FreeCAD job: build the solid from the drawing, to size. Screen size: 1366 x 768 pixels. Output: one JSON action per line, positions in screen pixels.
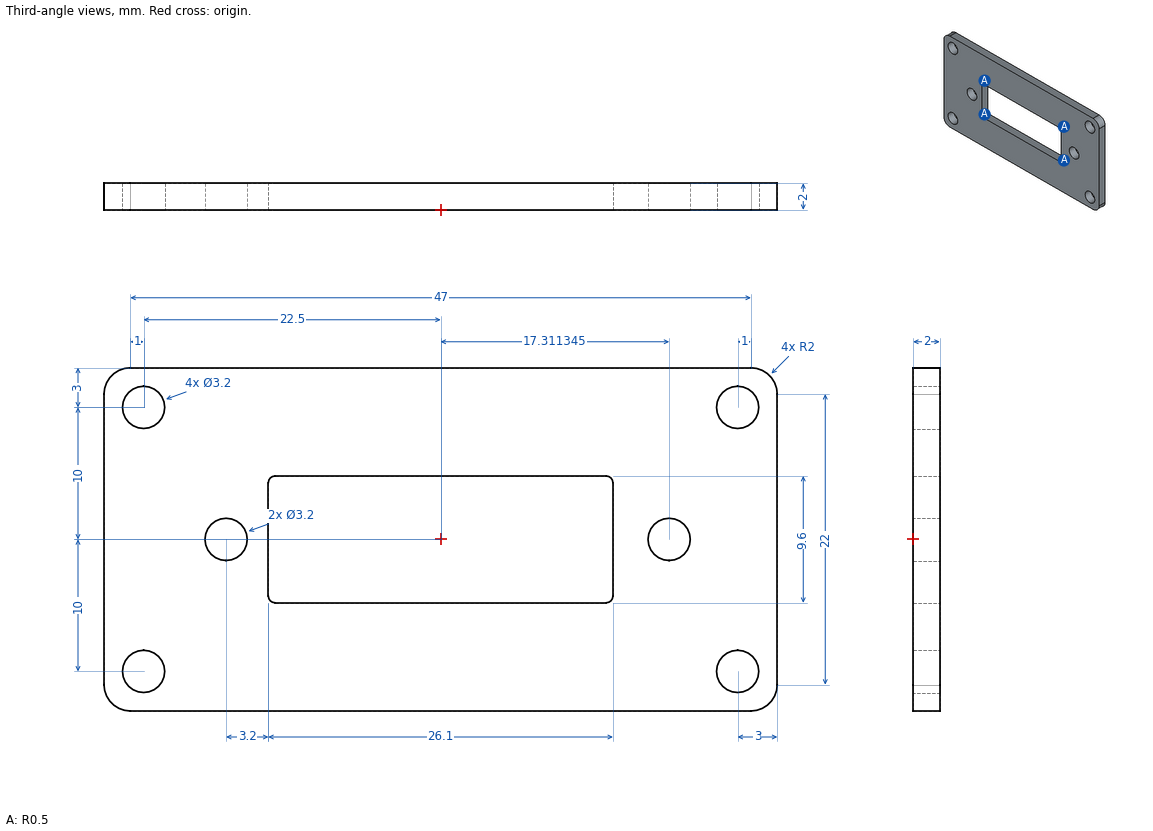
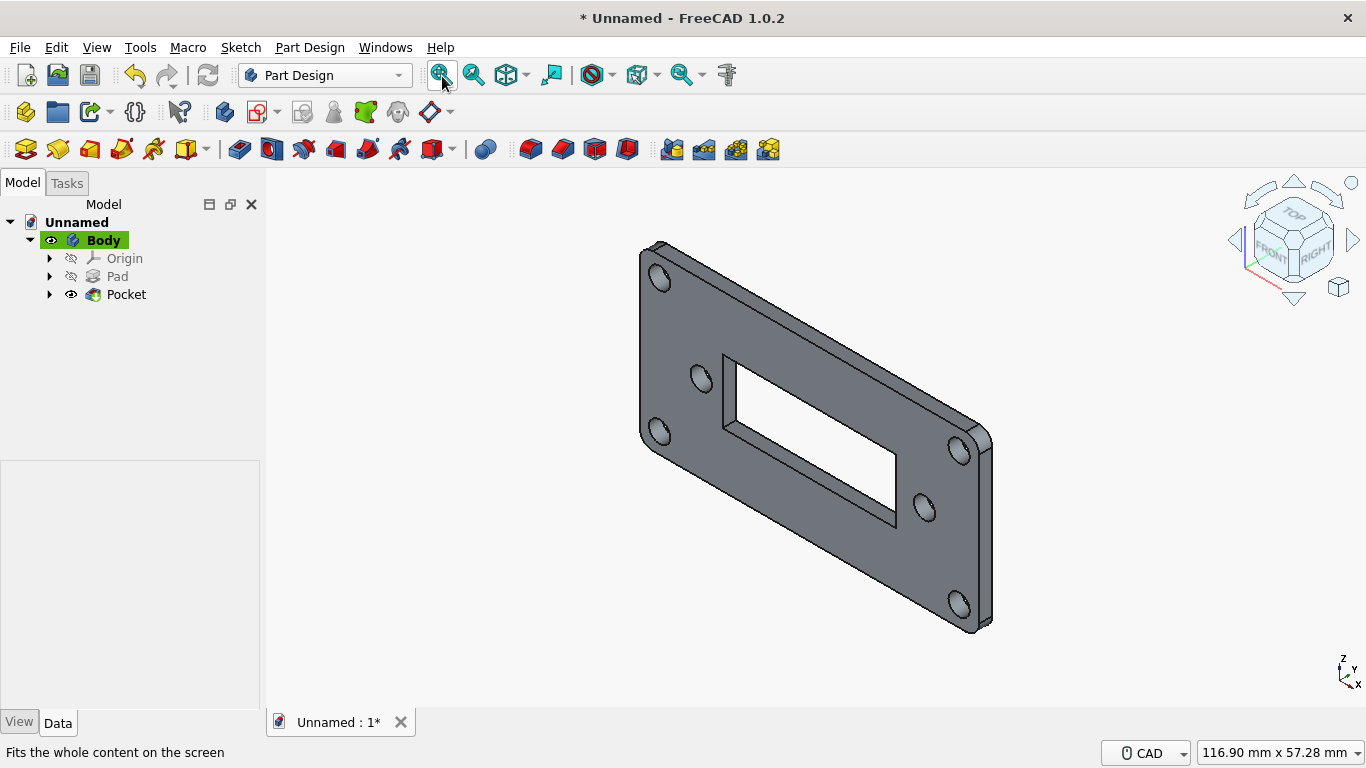
{"action": "scroll", "coordinate": [903, 450], "scroll_direction": "up", "scroll_amount": 4}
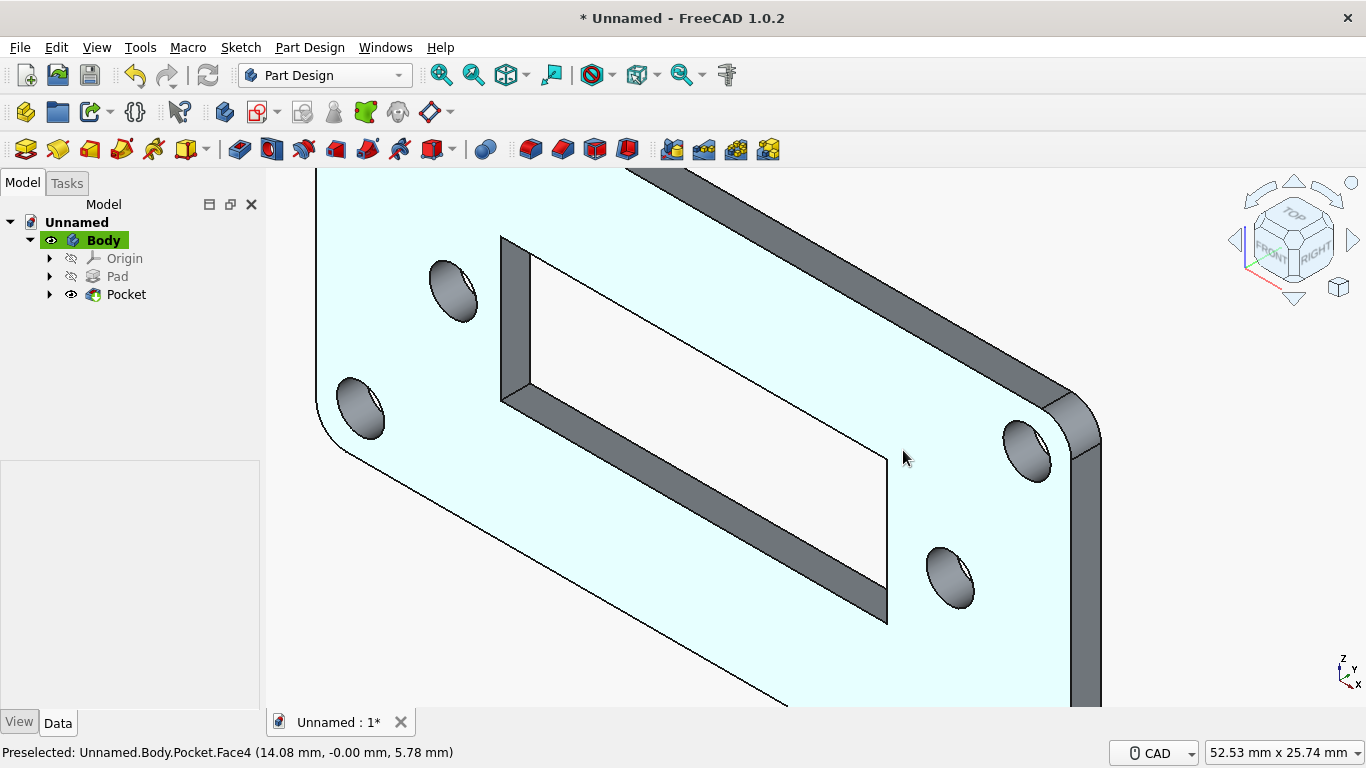
{"action": "left_click", "coordinate": [442, 76]}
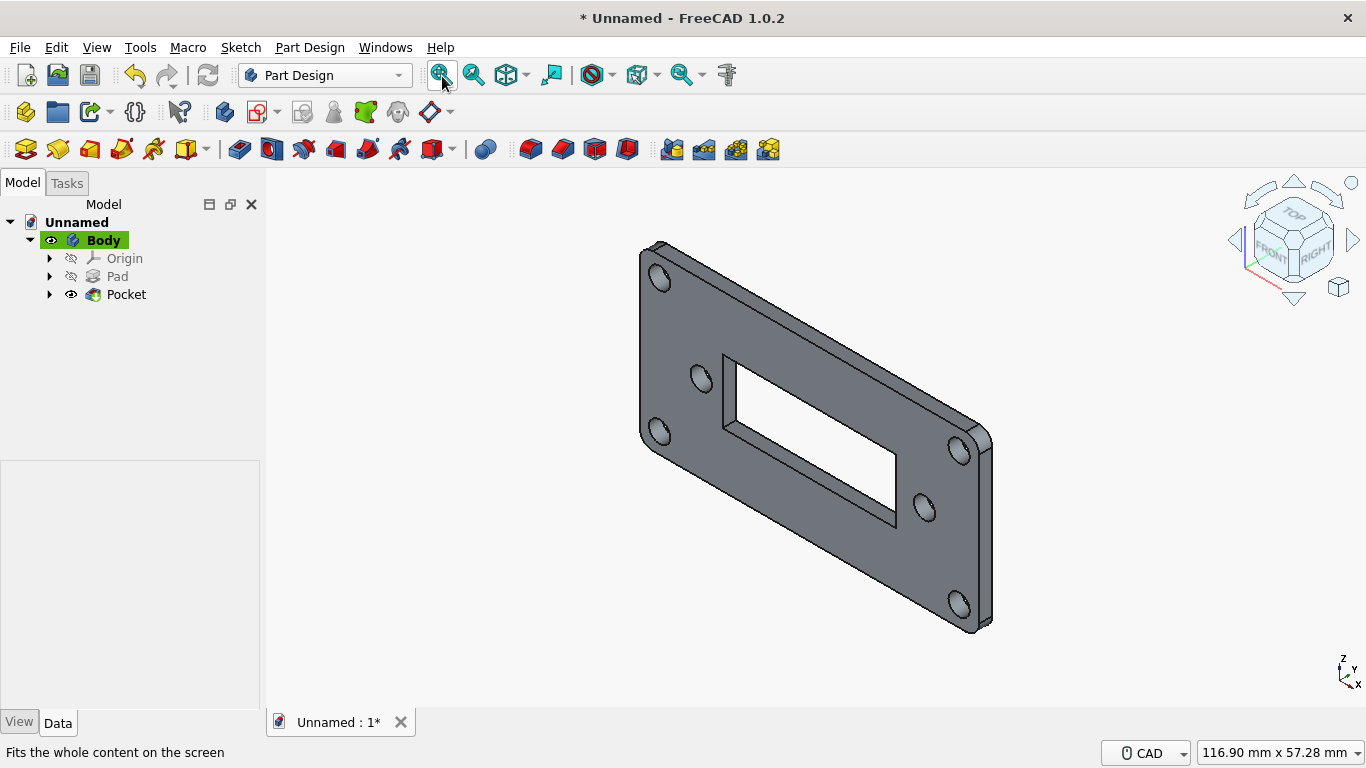
{"action": "key", "text": "2"}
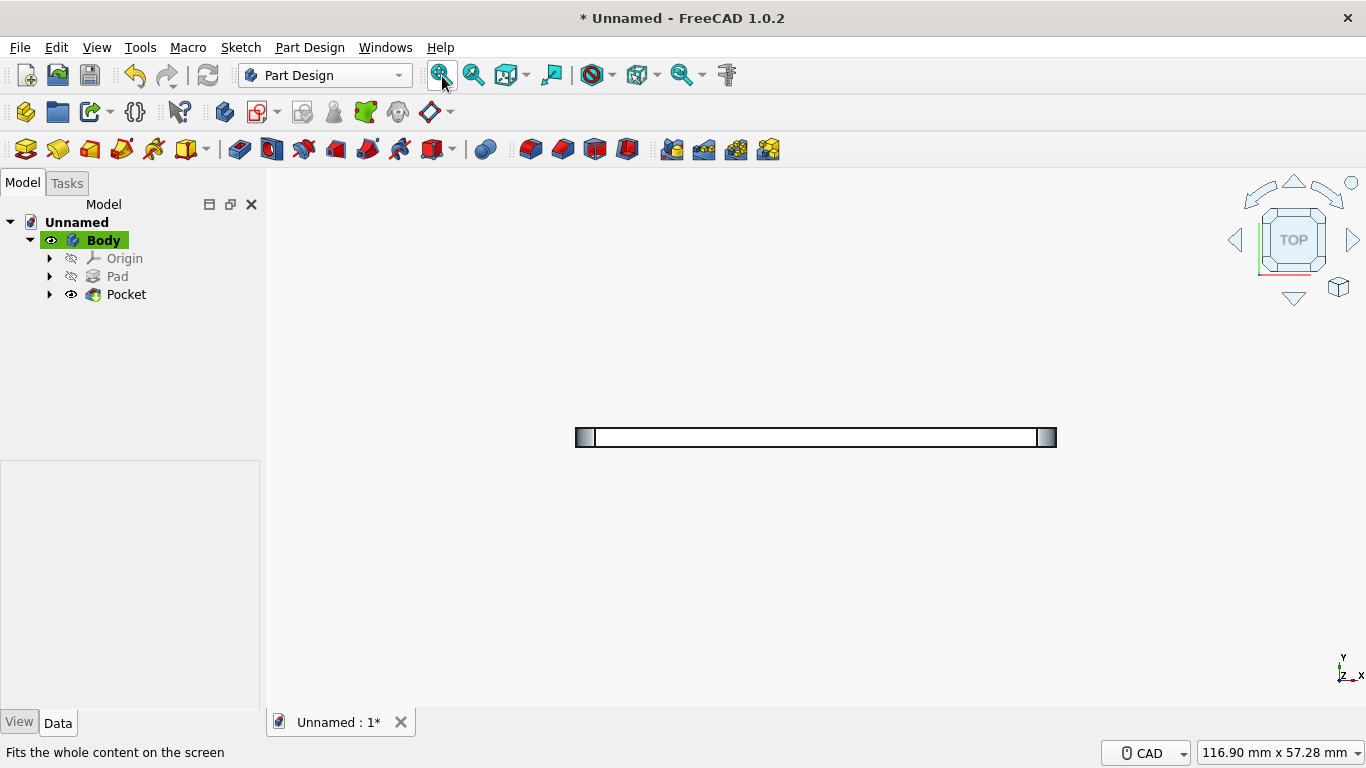
{"action": "left_click", "coordinate": [442, 76]}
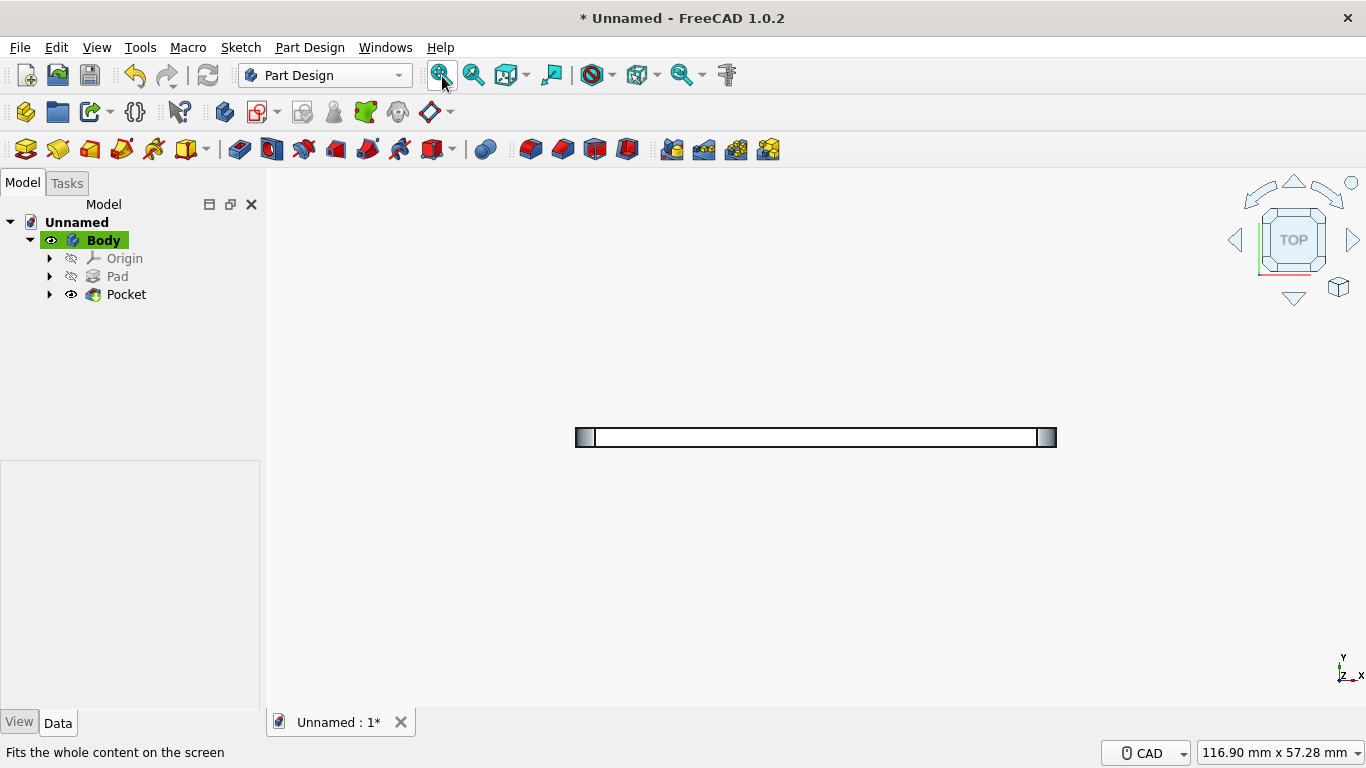
{"action": "scroll", "coordinate": [939, 436], "scroll_direction": "up", "scroll_amount": 4}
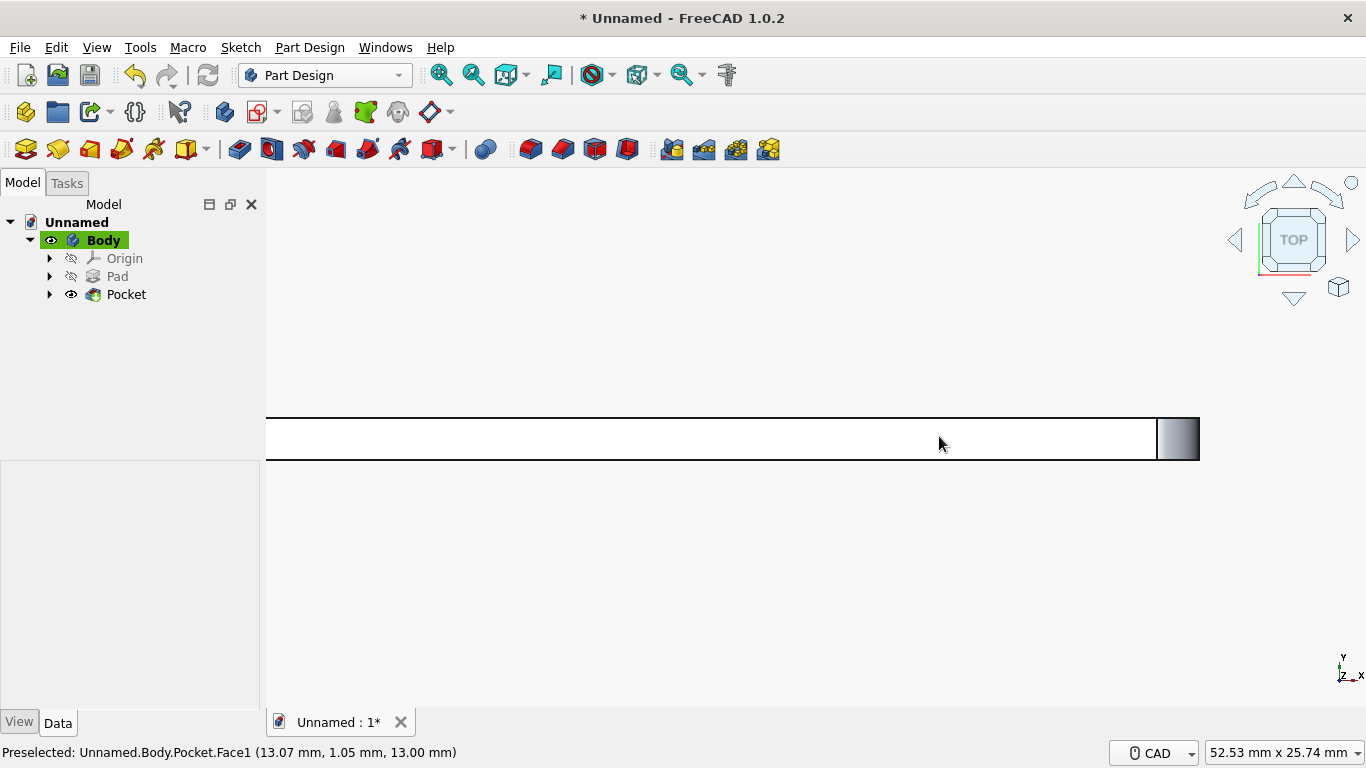
{"action": "left_click", "coordinate": [442, 76]}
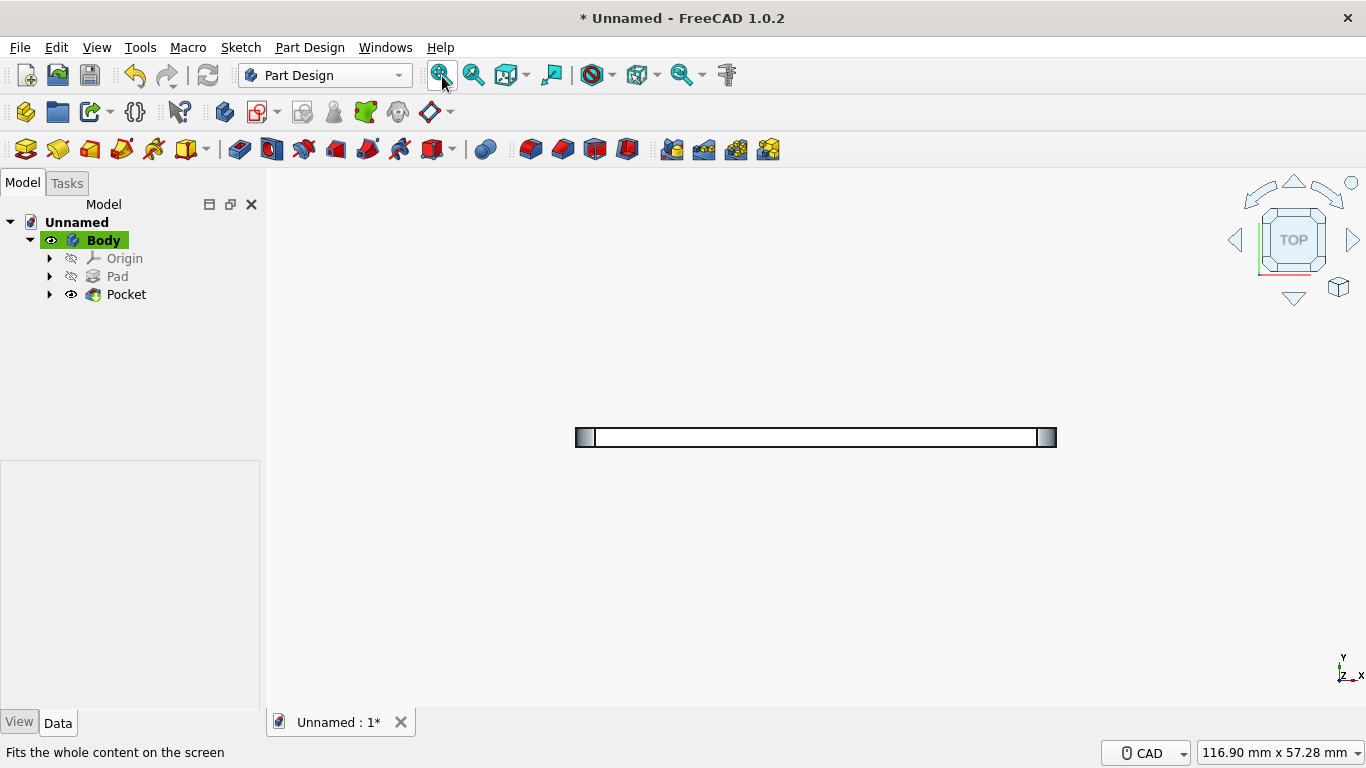
{"action": "key", "text": "1"}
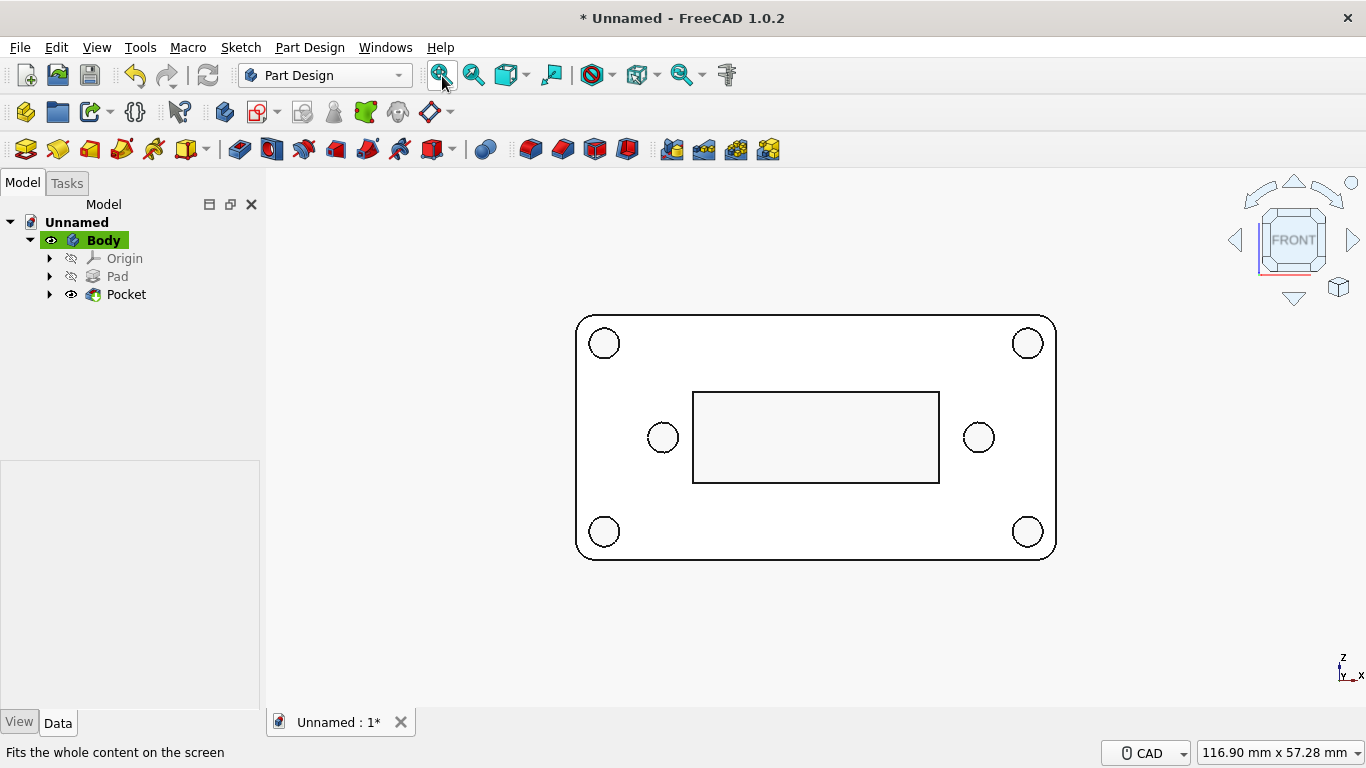
{"action": "scroll", "coordinate": [939, 391], "scroll_direction": "up", "scroll_amount": 4}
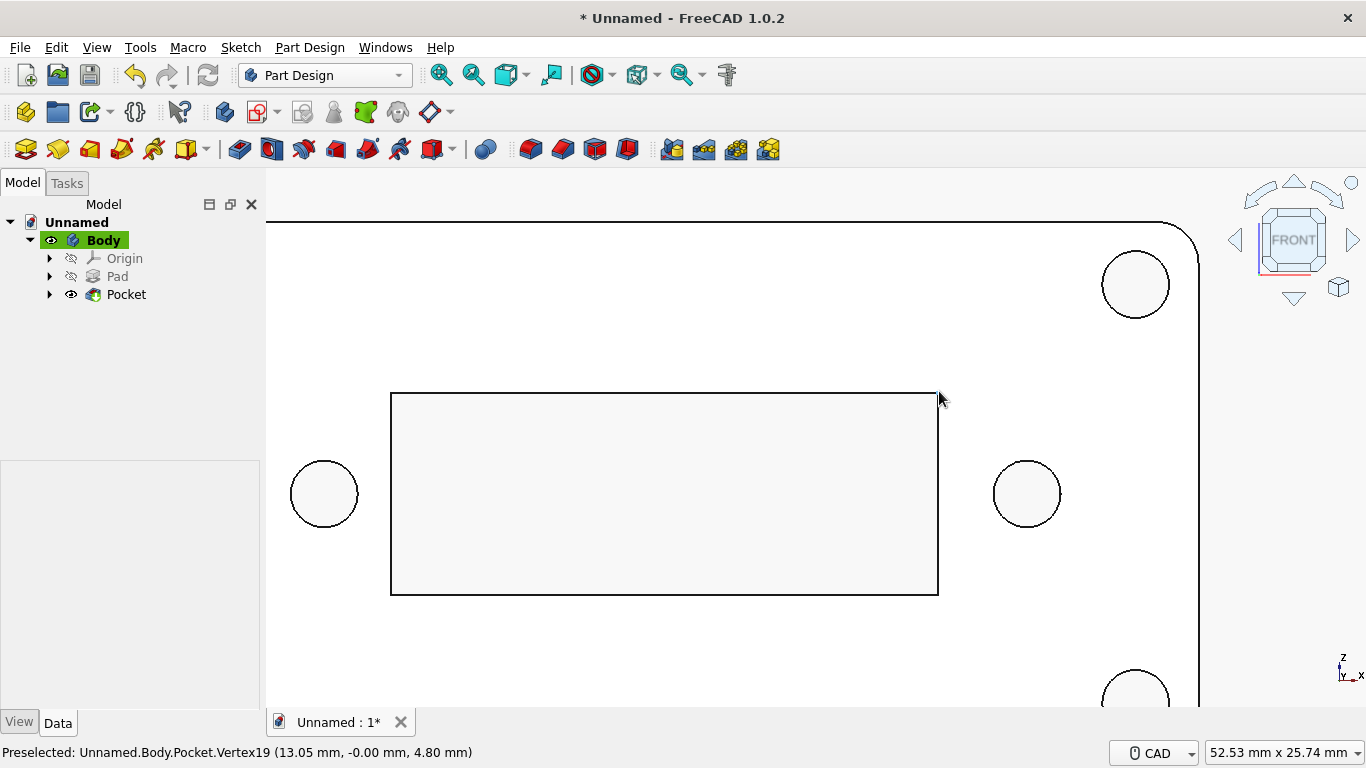
{"action": "left_click", "coordinate": [442, 76]}